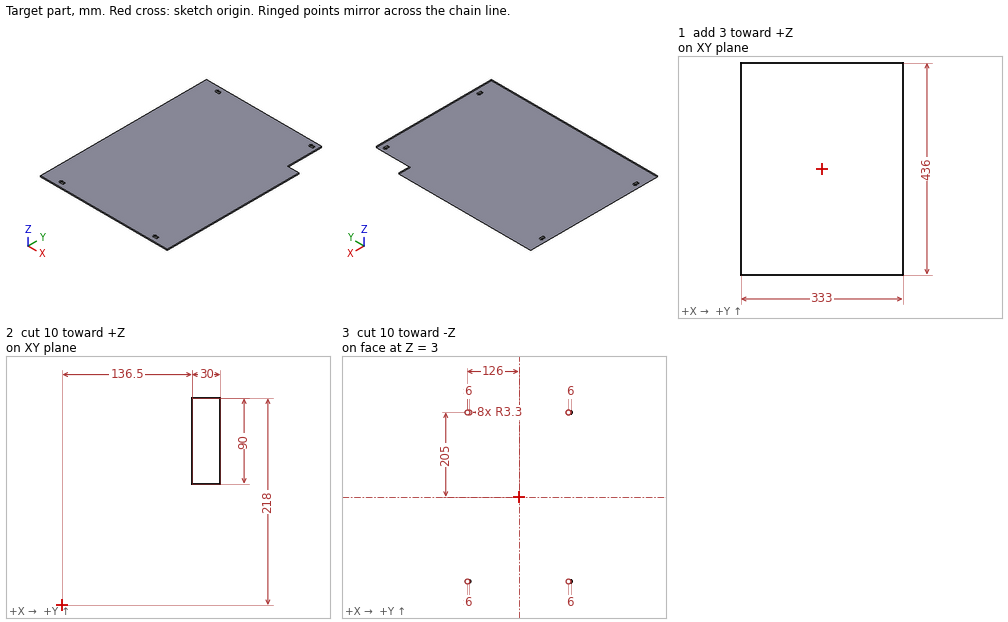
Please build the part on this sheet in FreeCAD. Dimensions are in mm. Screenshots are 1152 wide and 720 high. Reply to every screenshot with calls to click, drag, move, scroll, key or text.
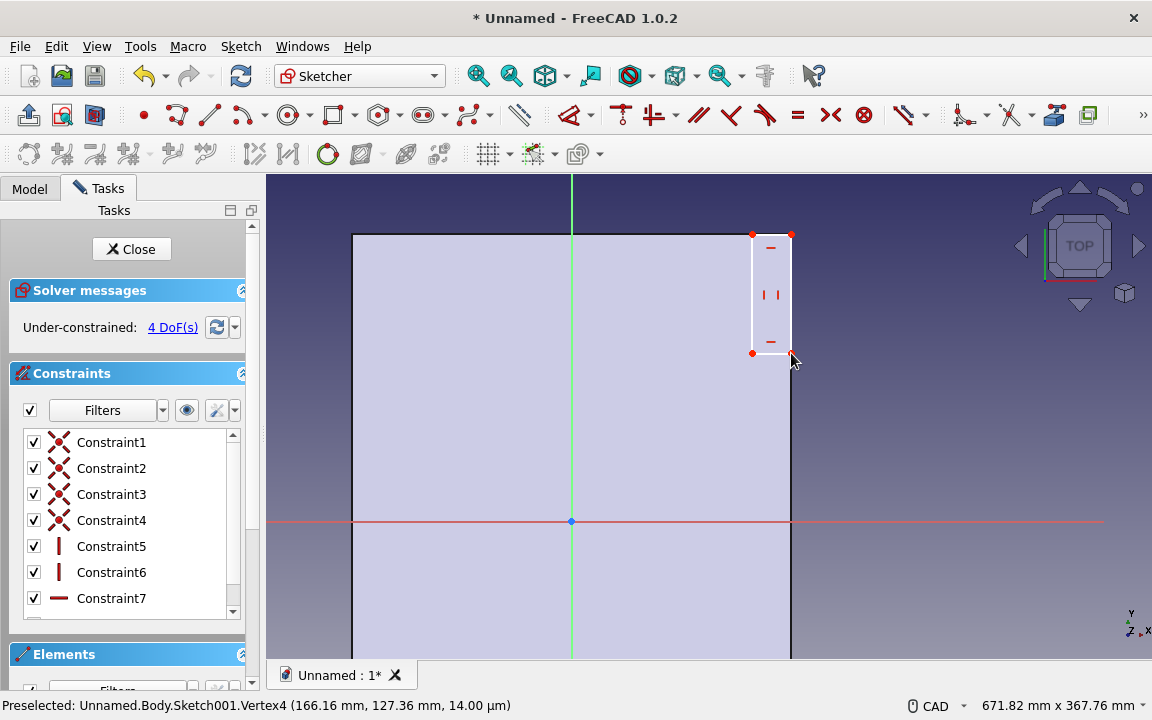
click(568, 116)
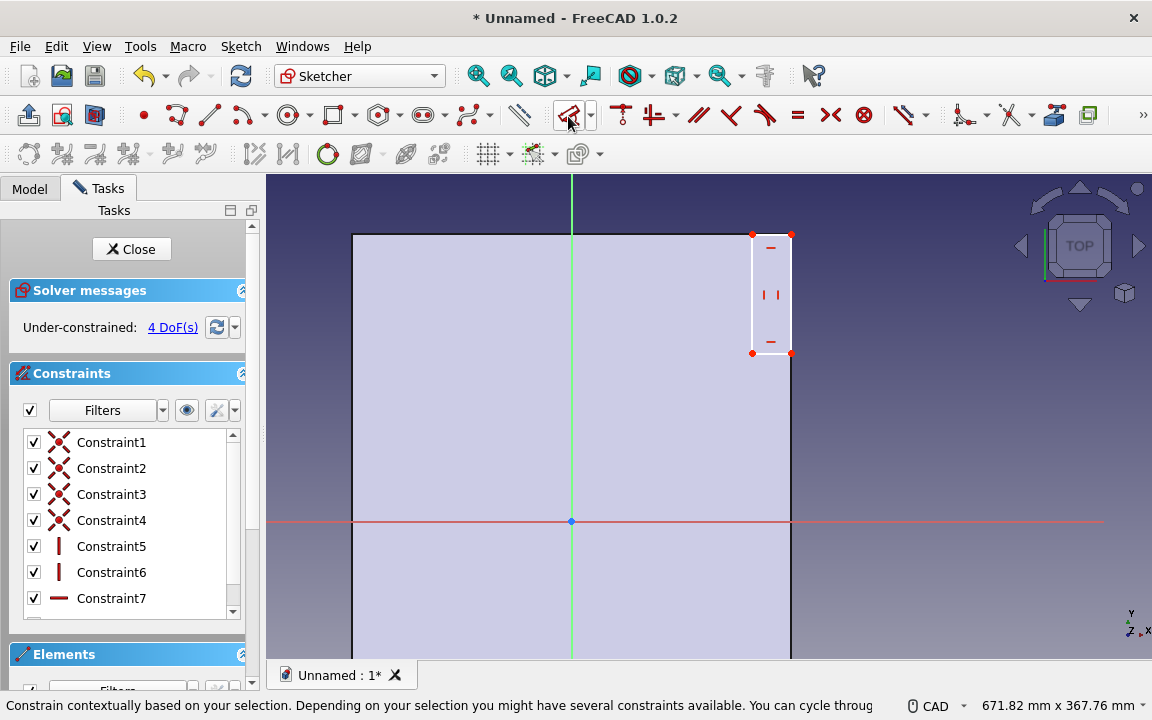
click(752, 271)
click(718, 295)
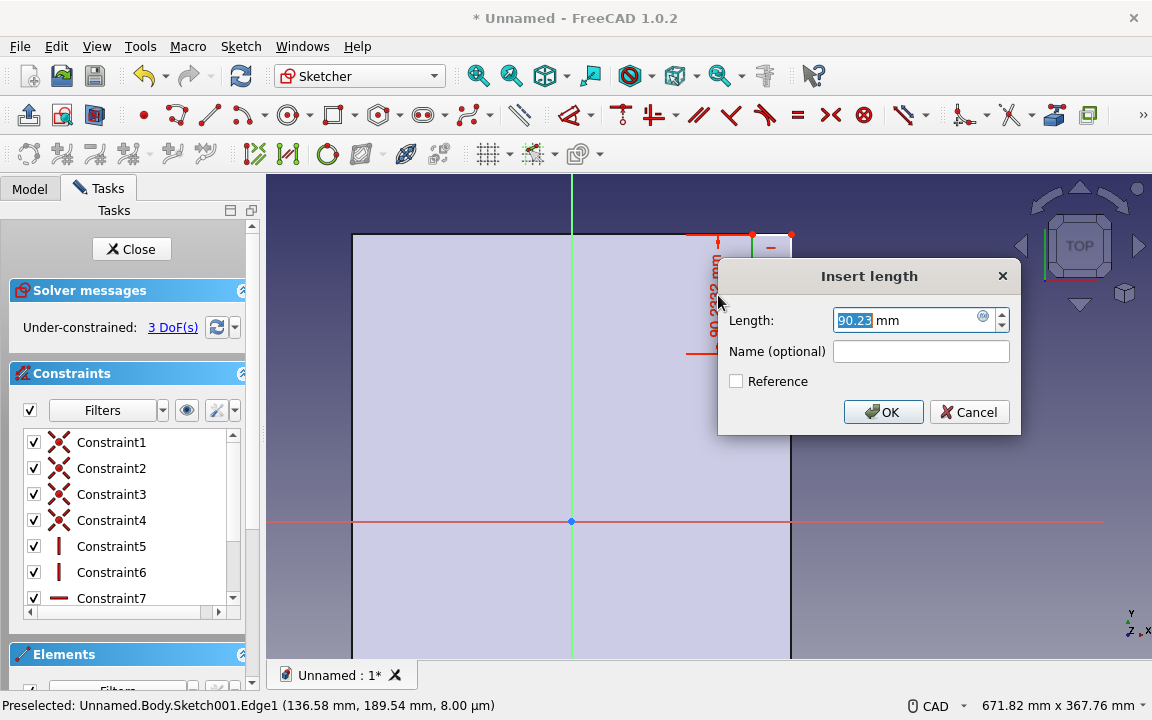
text(90)
key(Return)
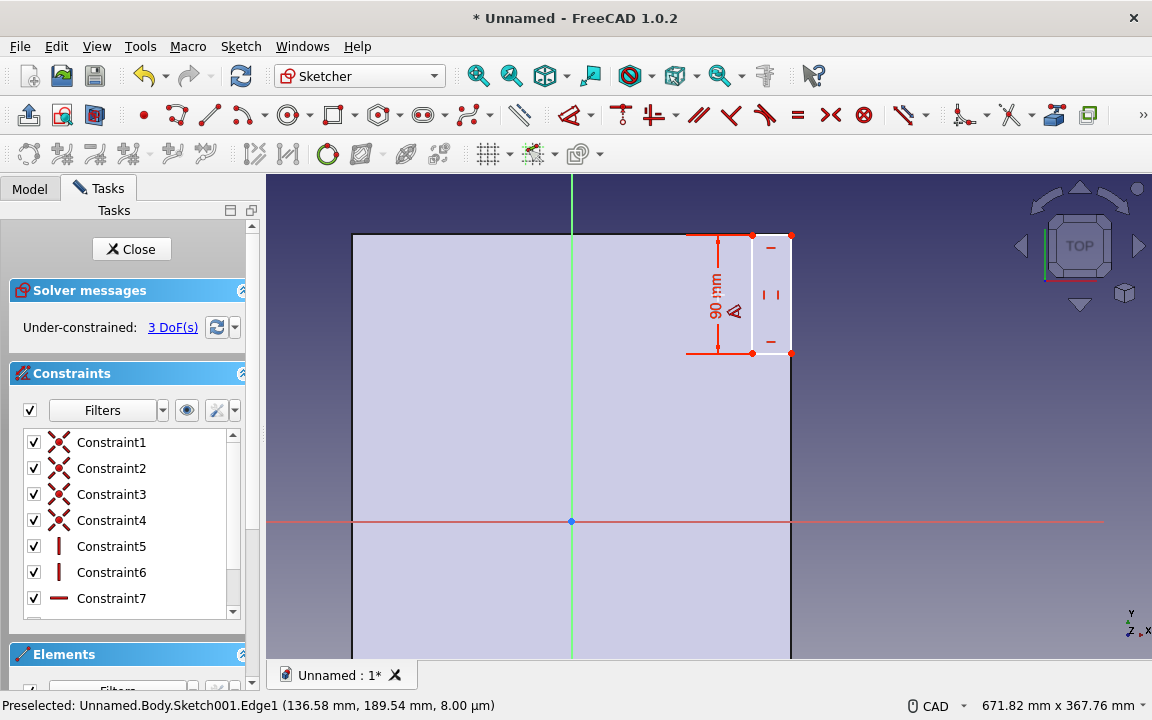
click(764, 354)
click(772, 320)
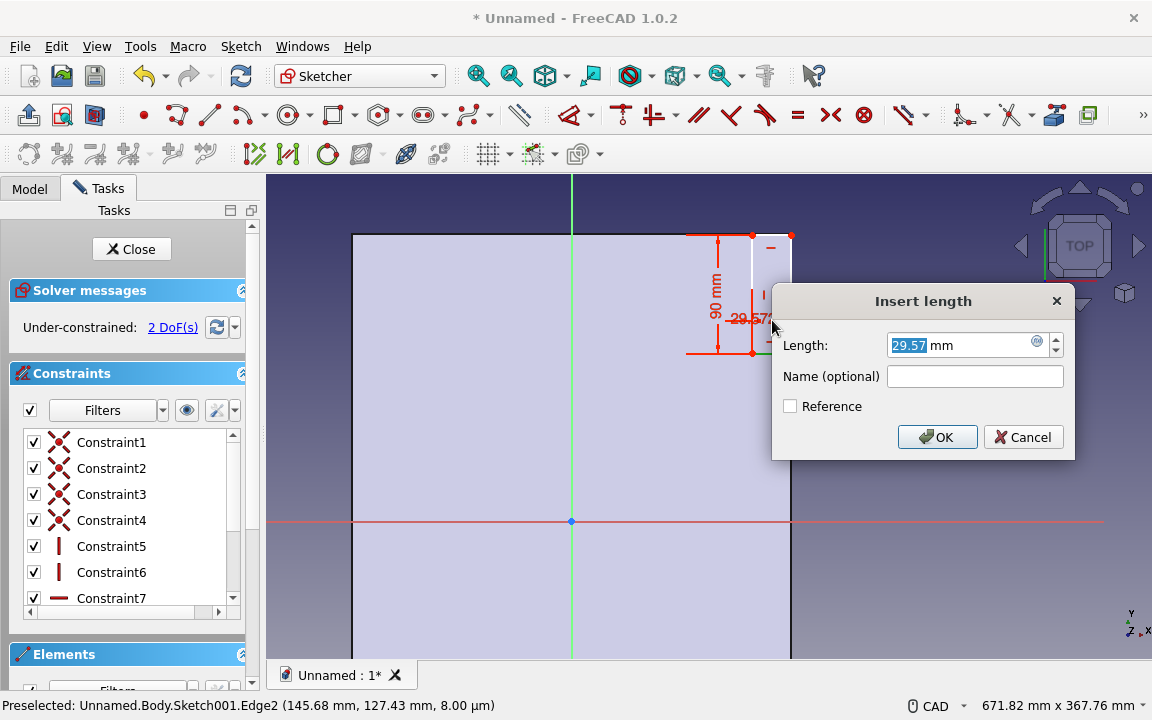
text(30)
key(Return)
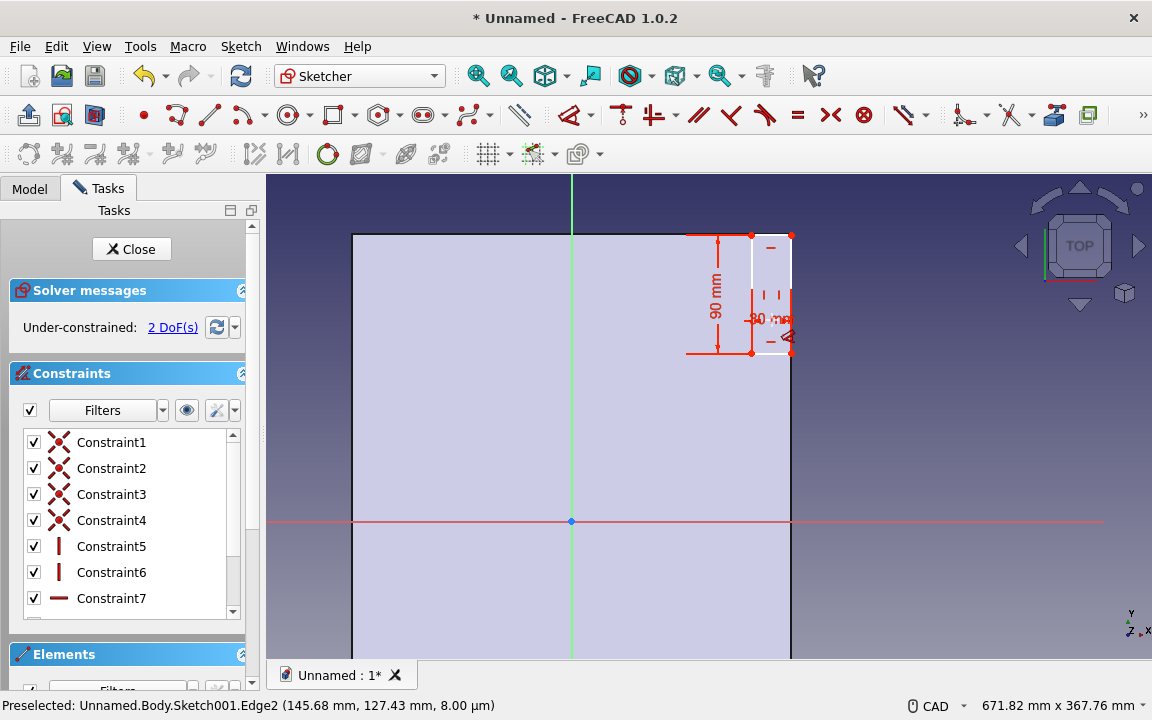
click(752, 235)
click(538, 379)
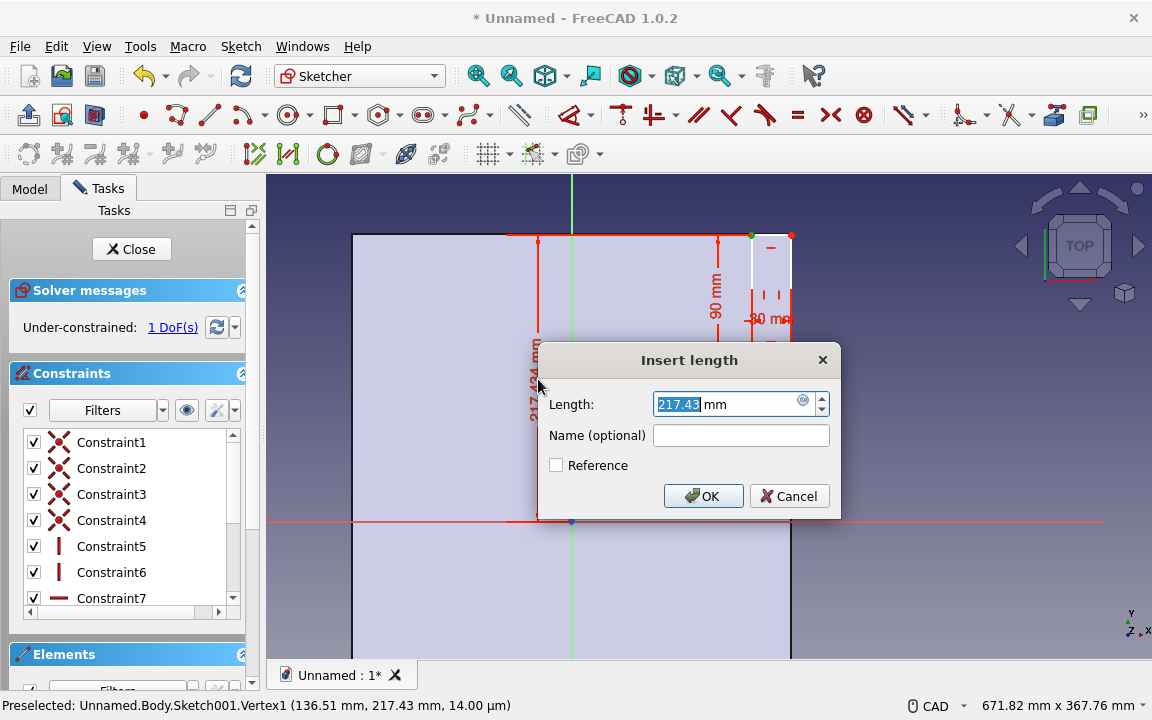
text(218)
key(Return)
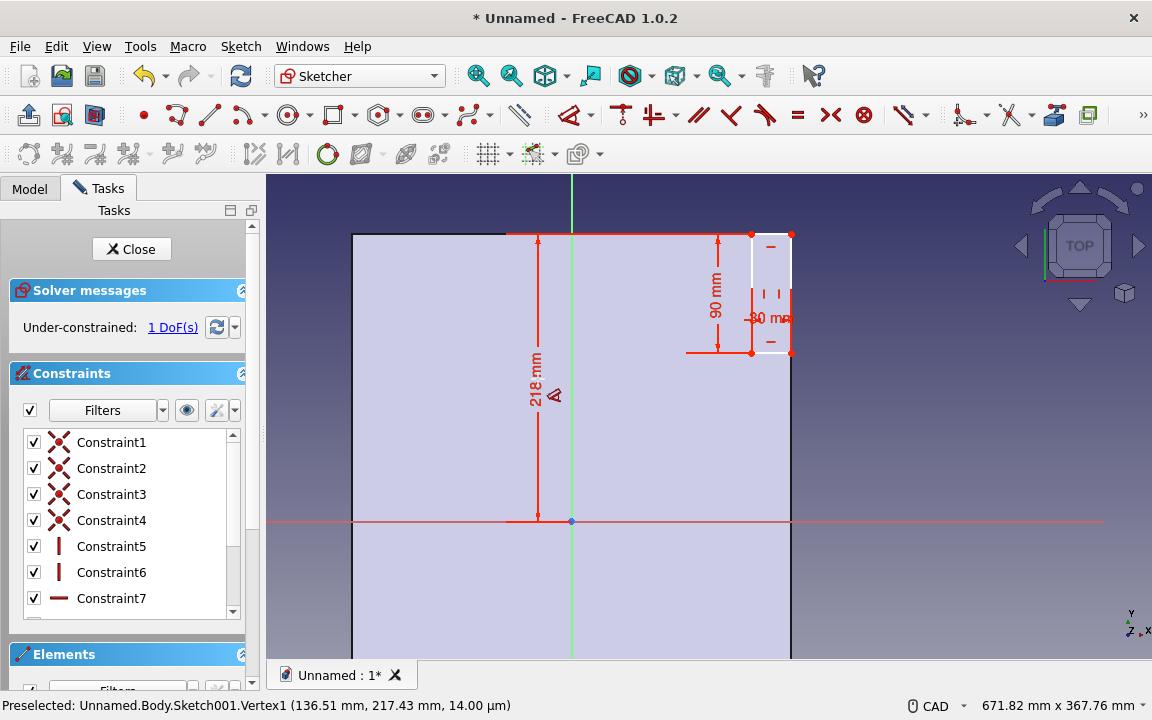
click(752, 234)
click(662, 556)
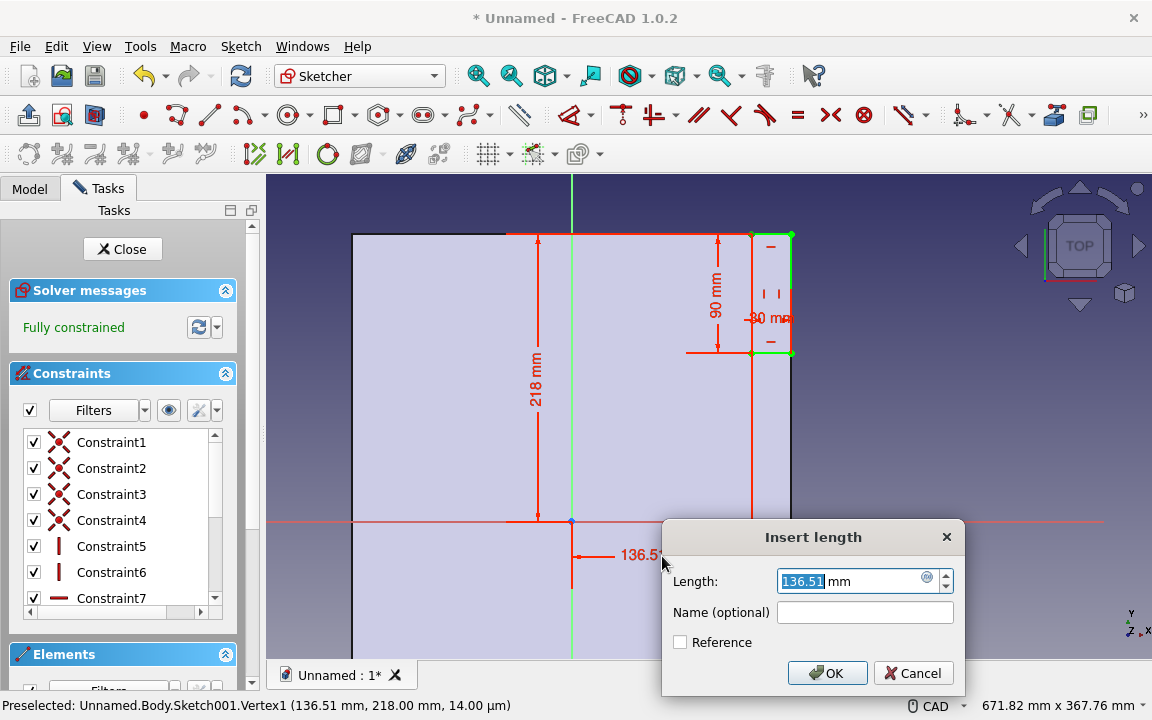
text(136.5)
key(Return)
key(Escape)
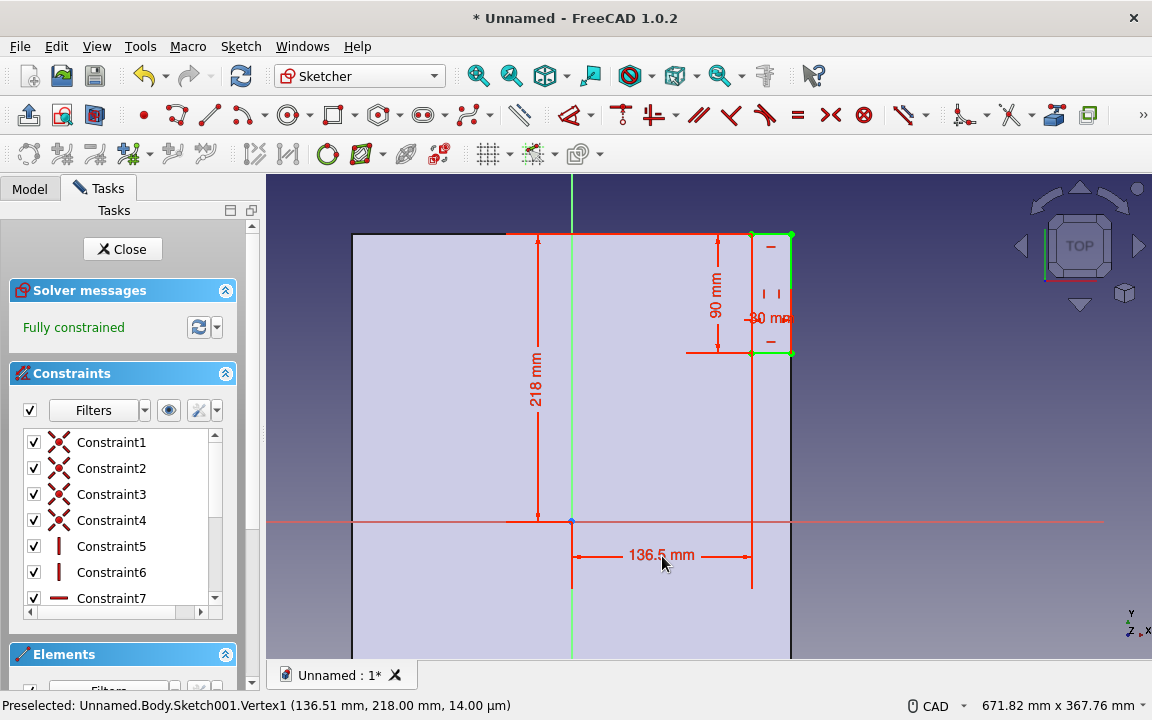
click(123, 249)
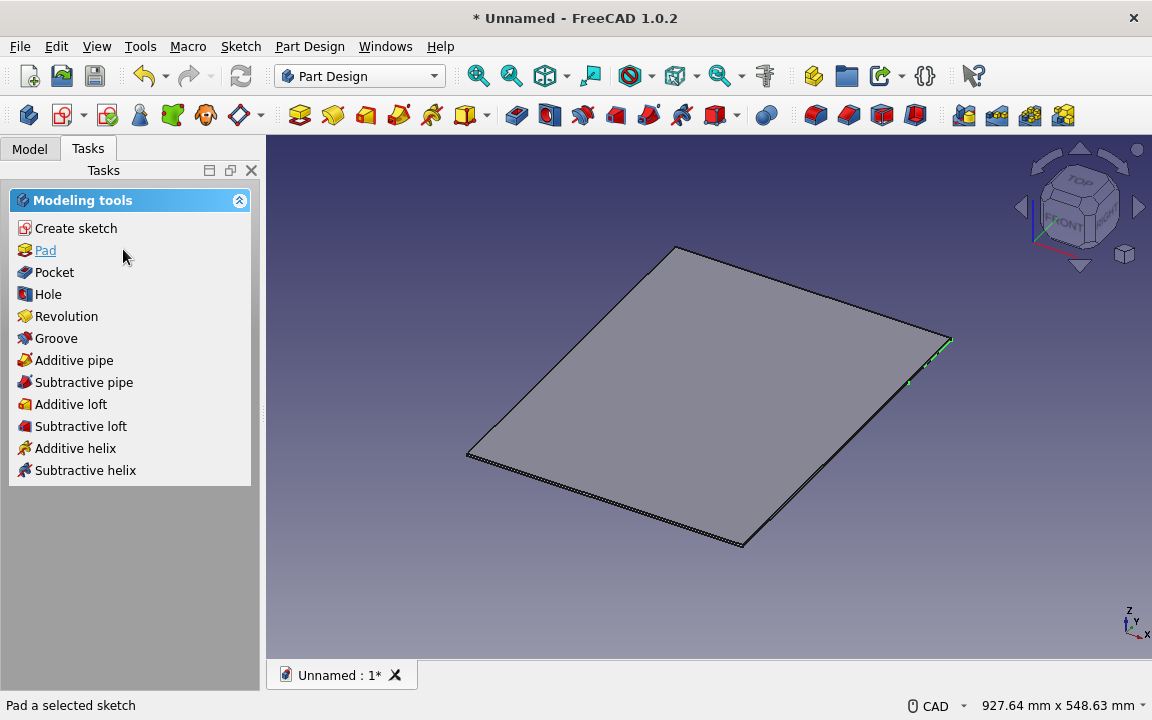
click(517, 116)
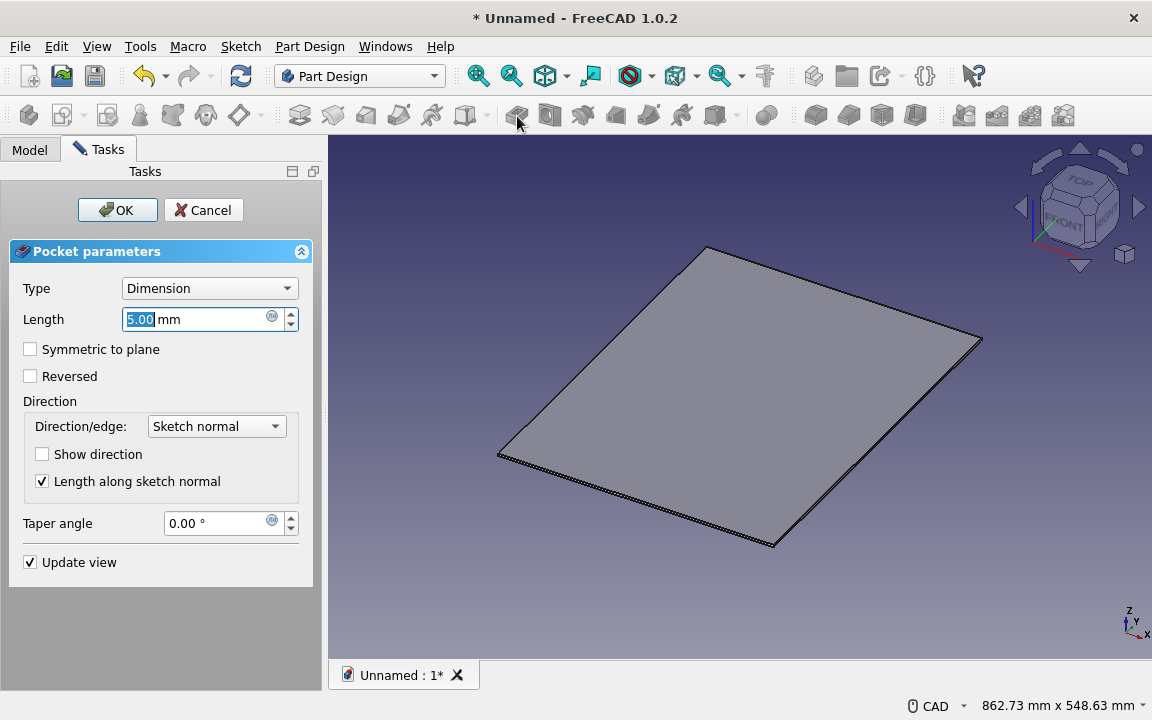
text(10)
key(Tab)